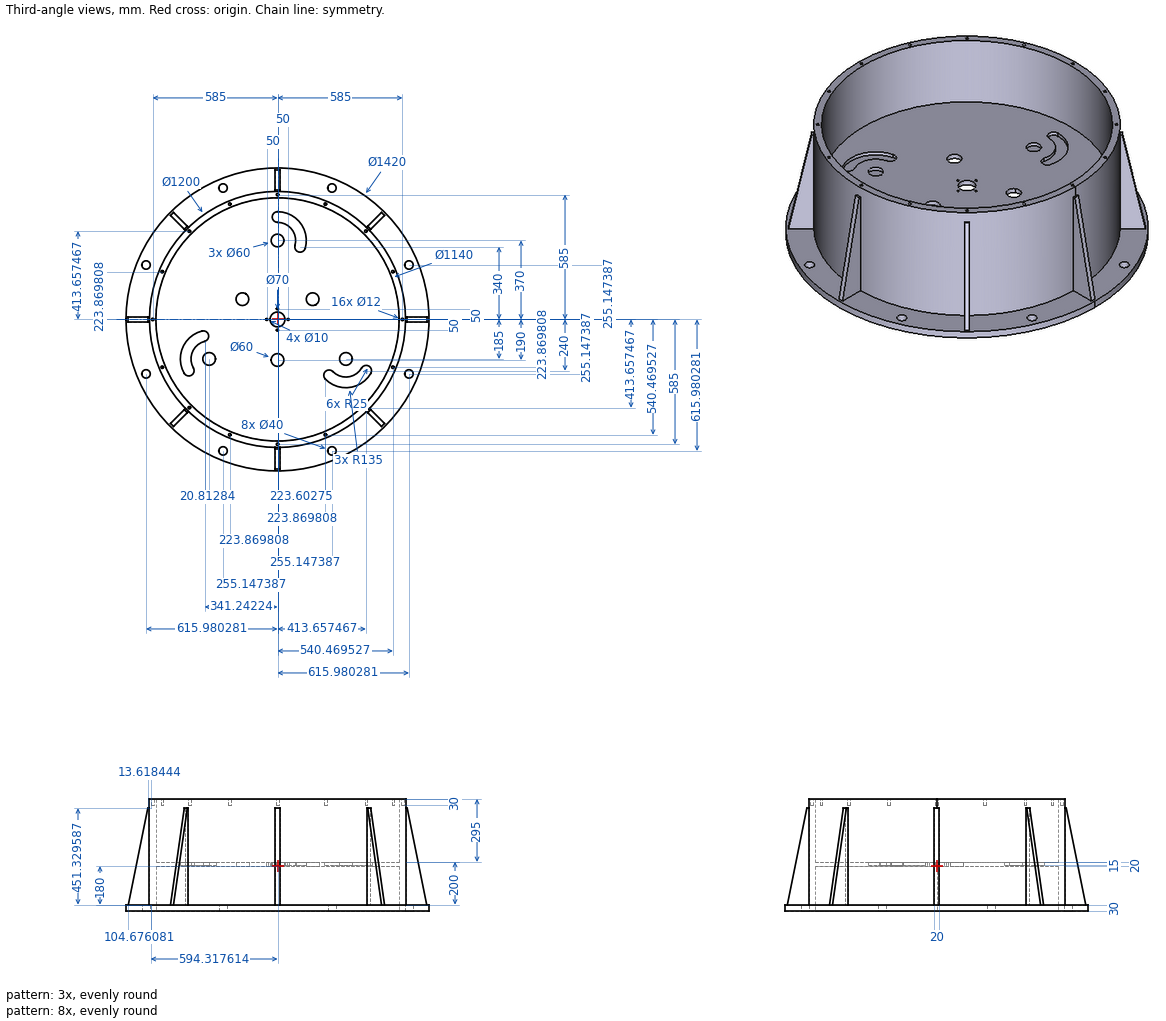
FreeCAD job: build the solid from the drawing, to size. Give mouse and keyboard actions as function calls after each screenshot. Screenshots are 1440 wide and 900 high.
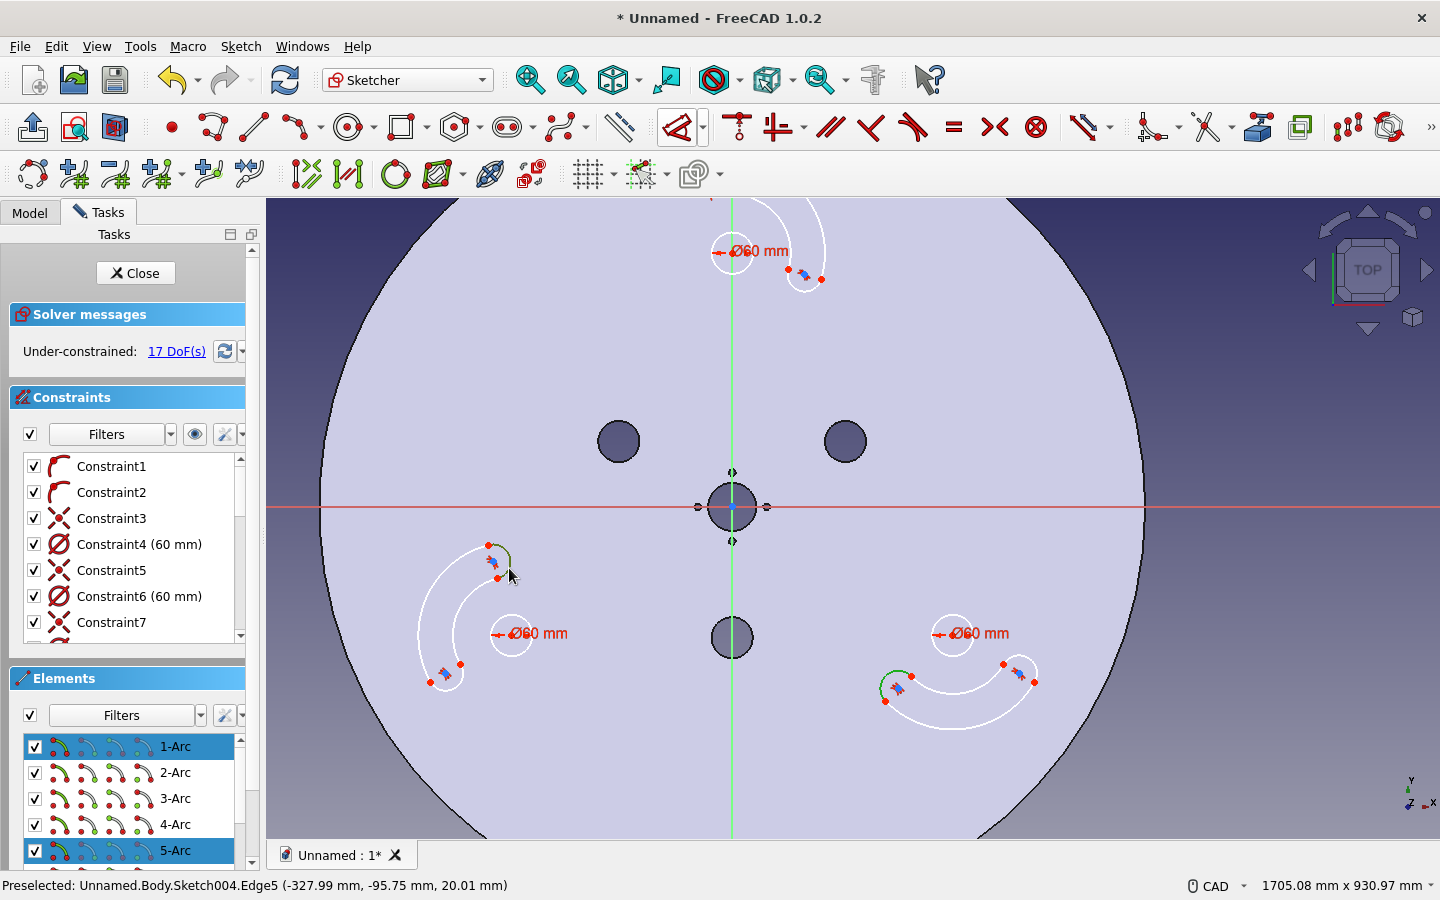
click(791, 285)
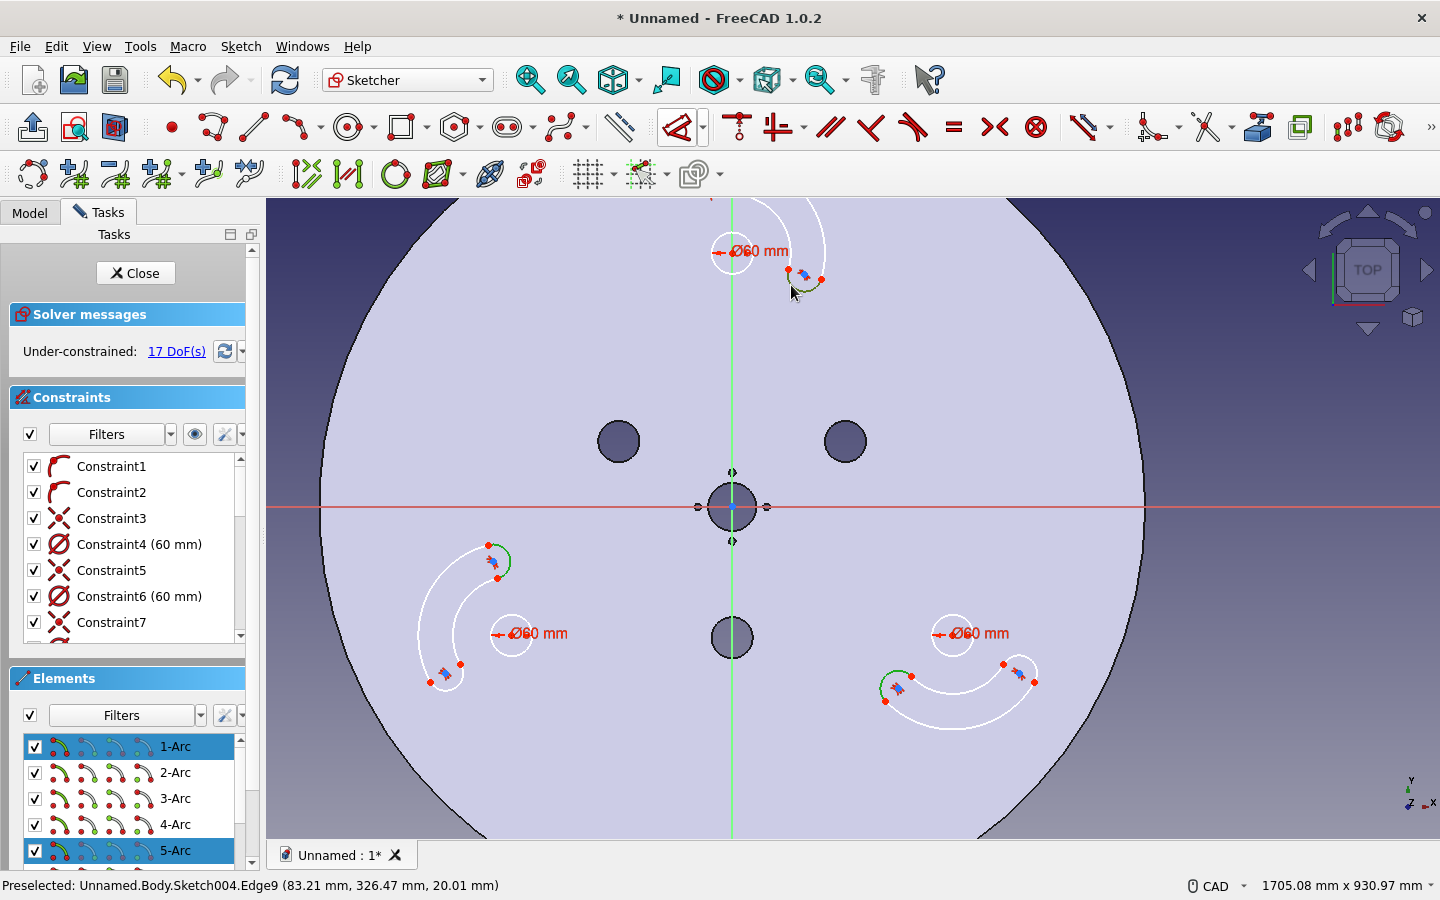
click(954, 128)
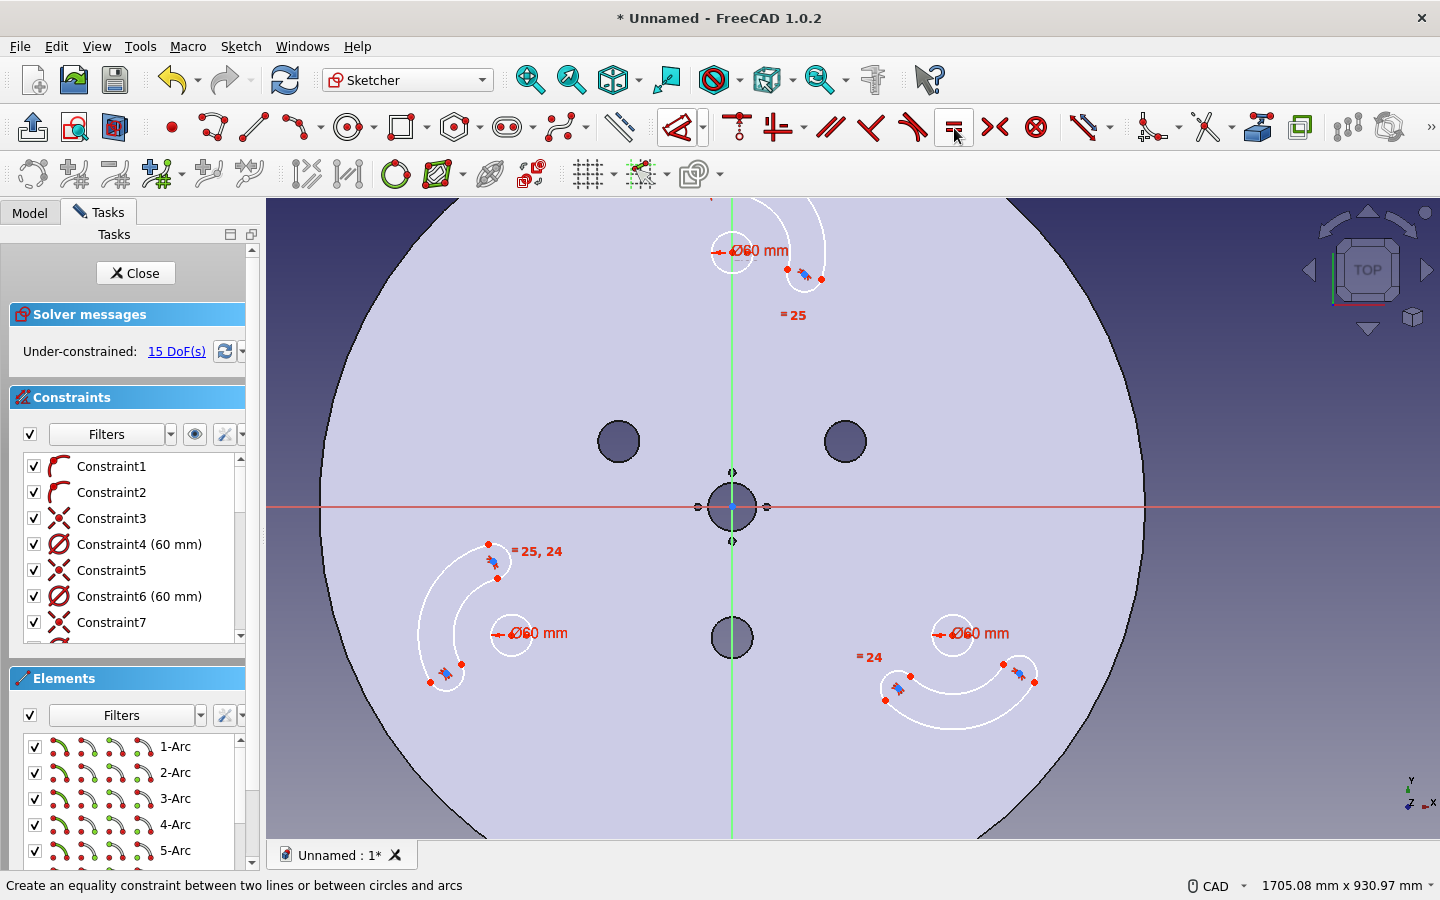
click(930, 727)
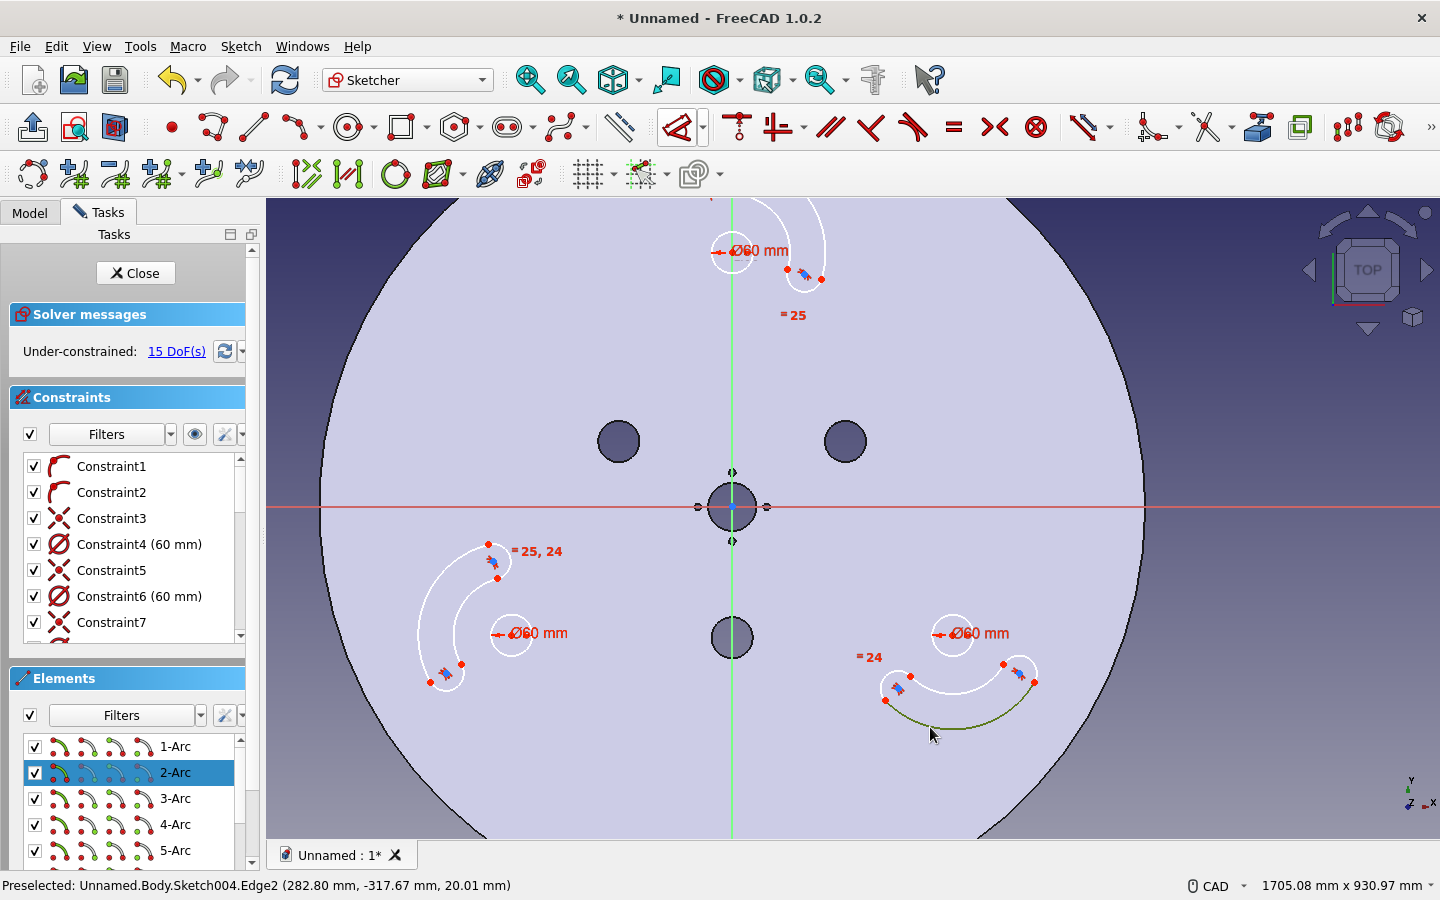
click(445, 570)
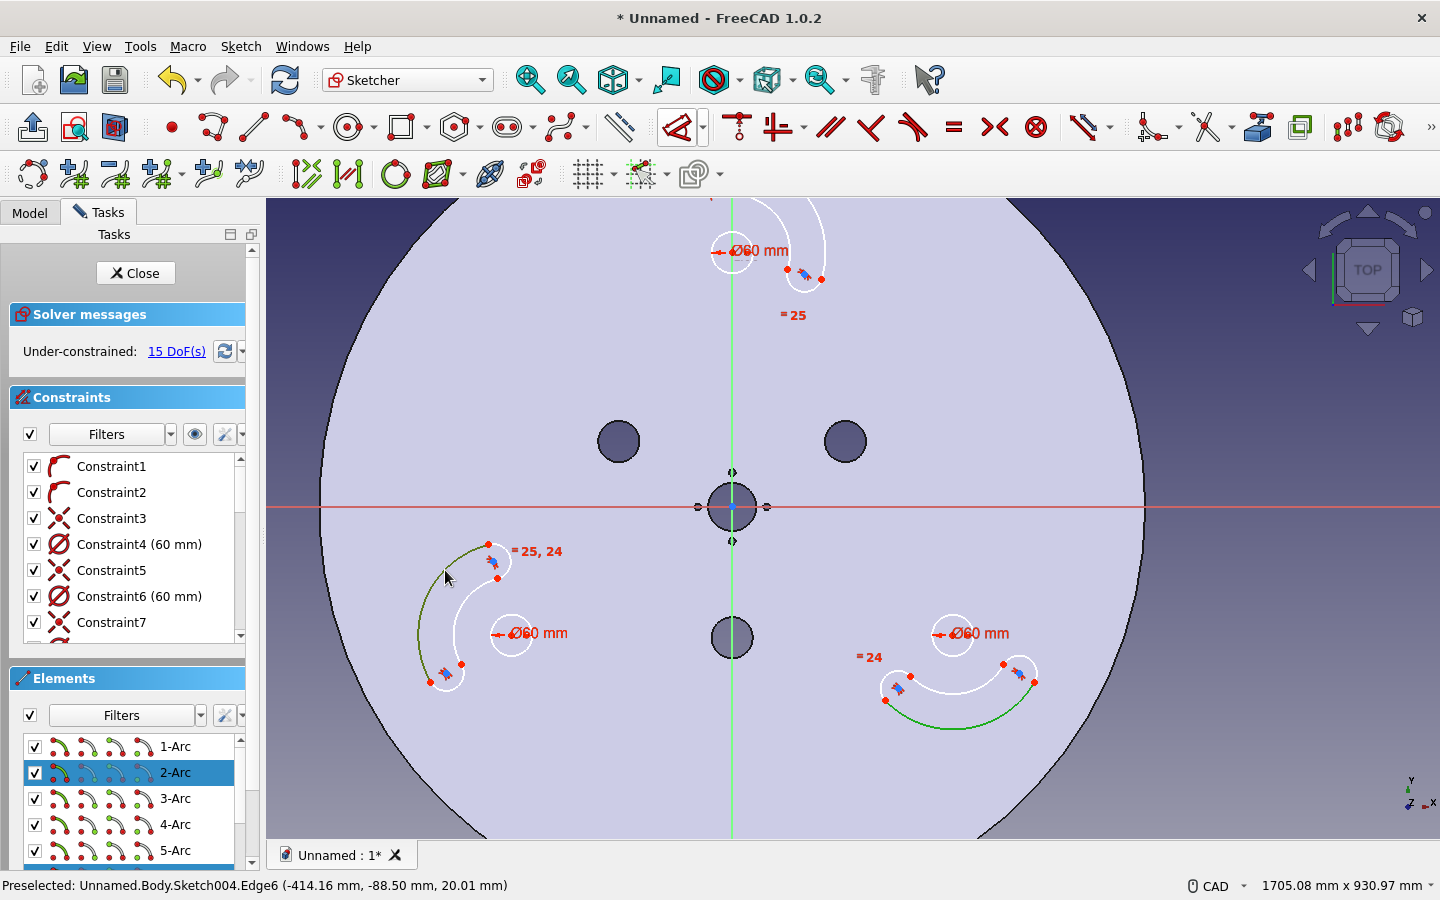
click(822, 228)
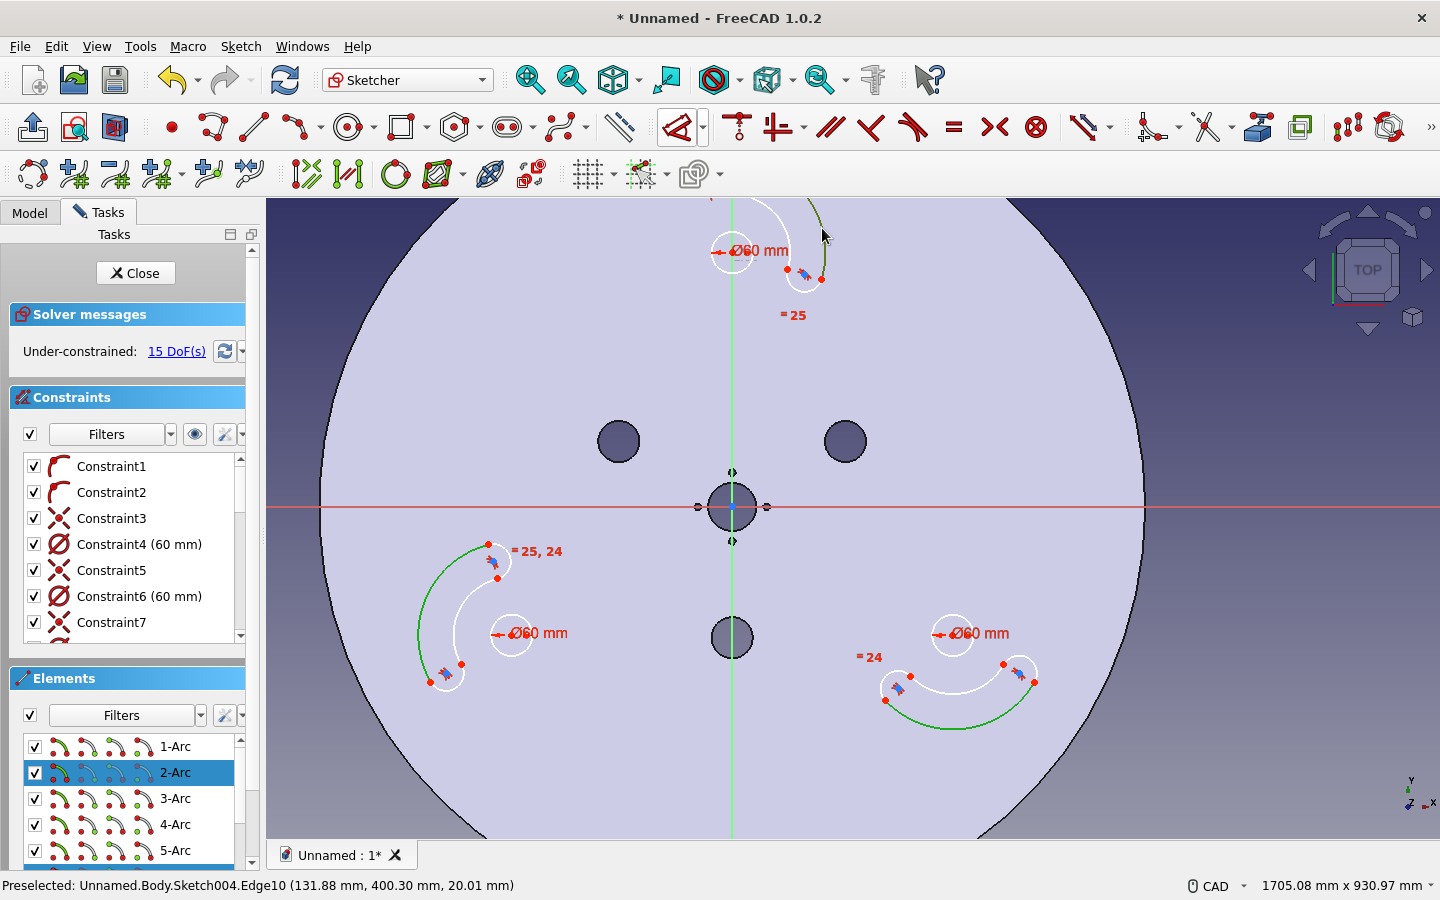
click(954, 128)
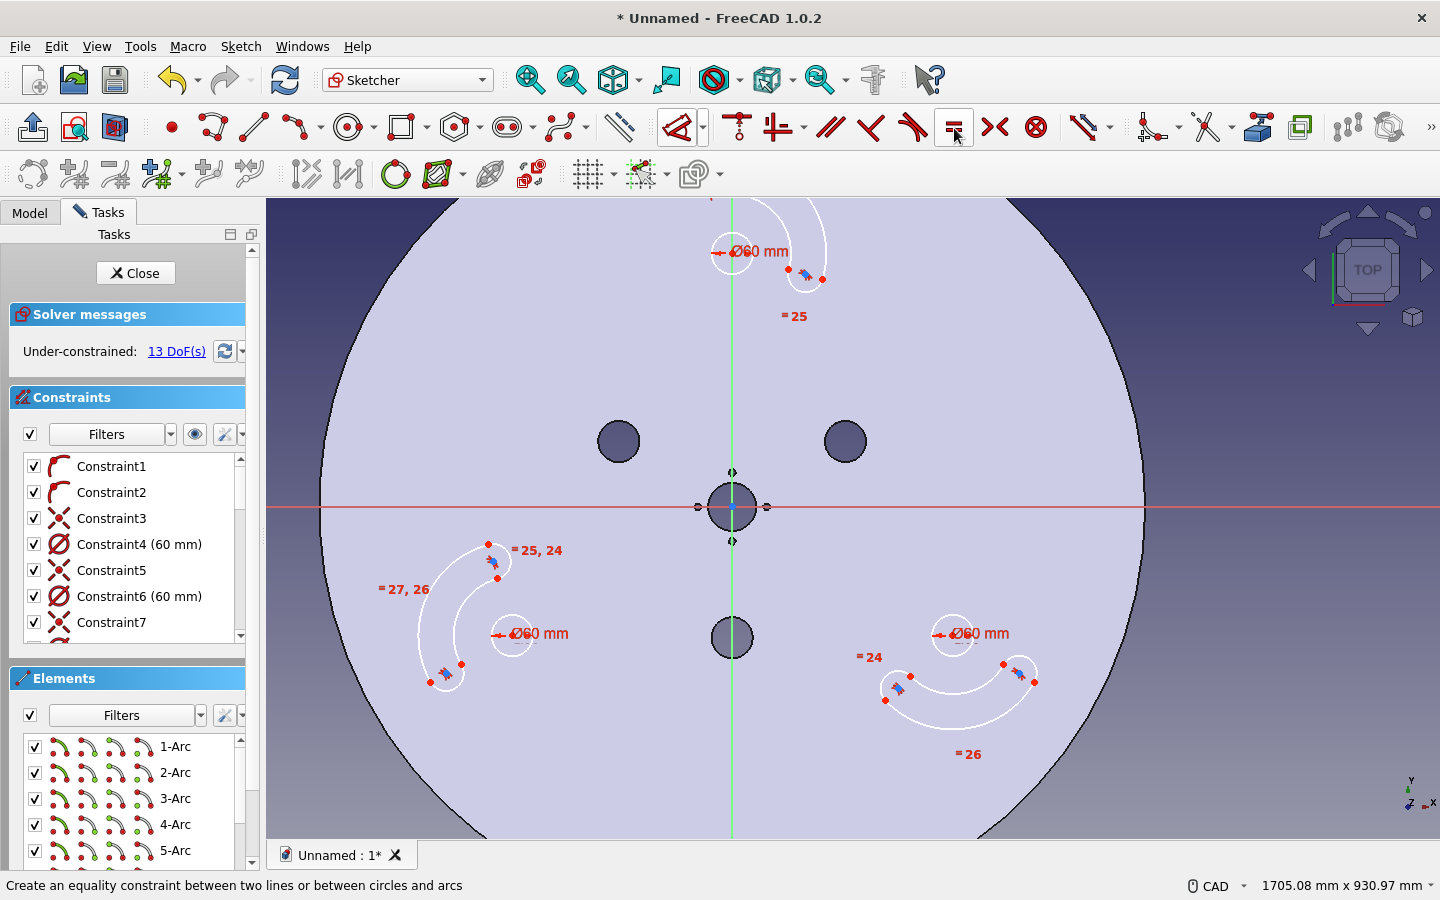
click(732, 253)